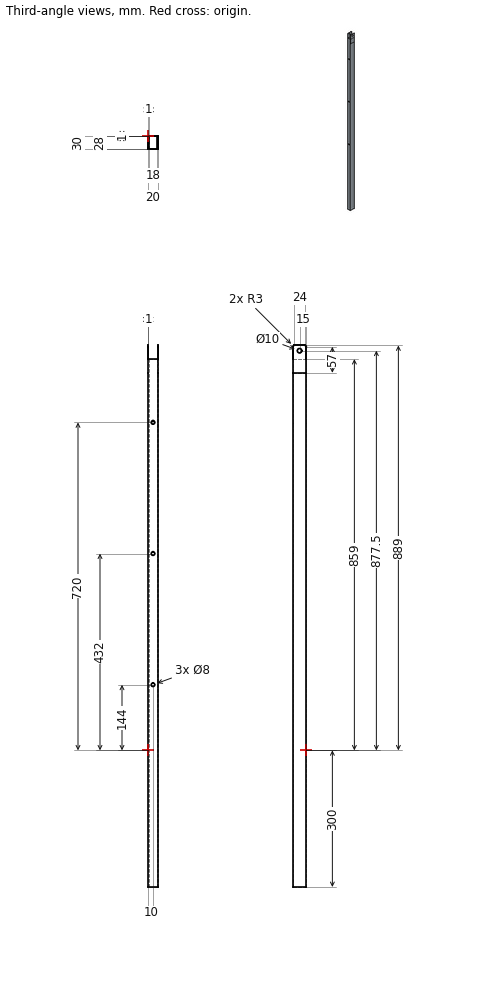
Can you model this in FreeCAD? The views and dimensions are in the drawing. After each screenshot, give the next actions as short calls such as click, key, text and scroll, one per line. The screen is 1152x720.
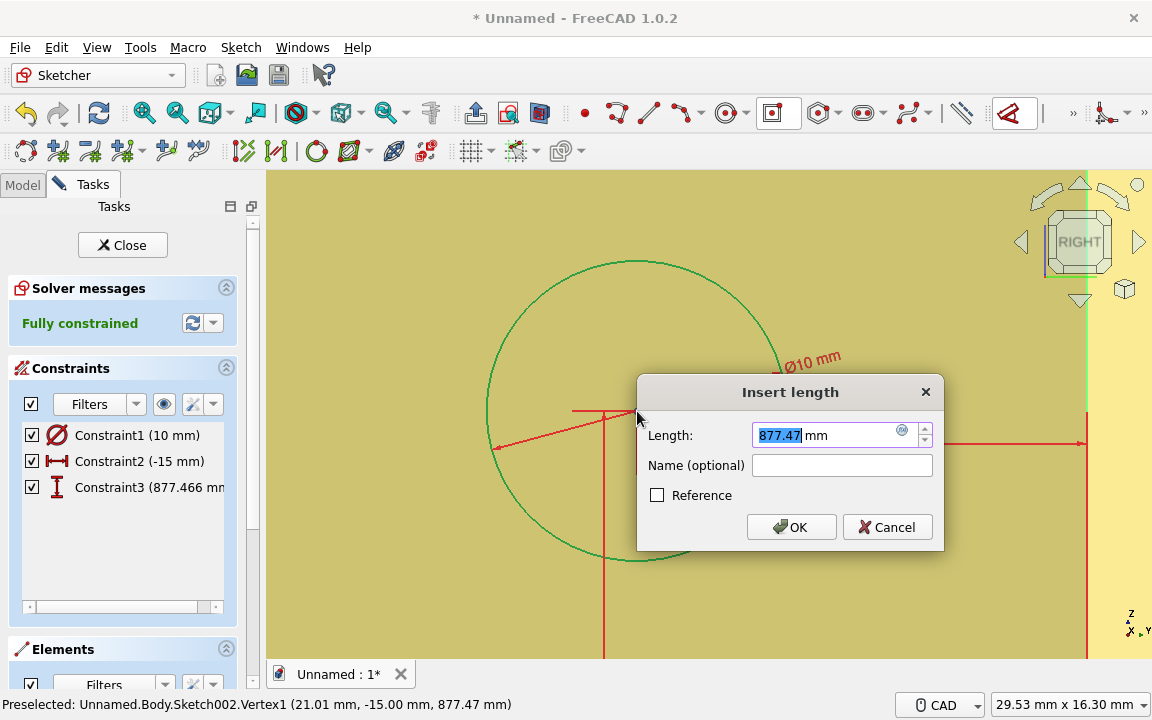
text(877.5)
key(Return)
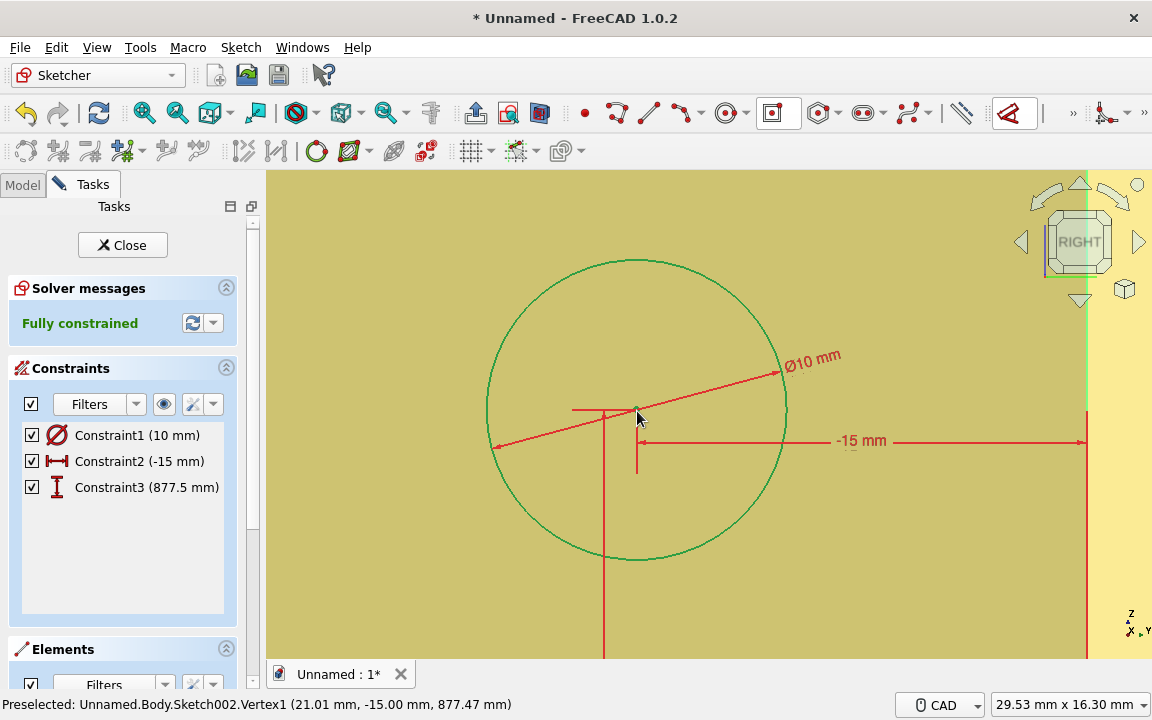
click(123, 245)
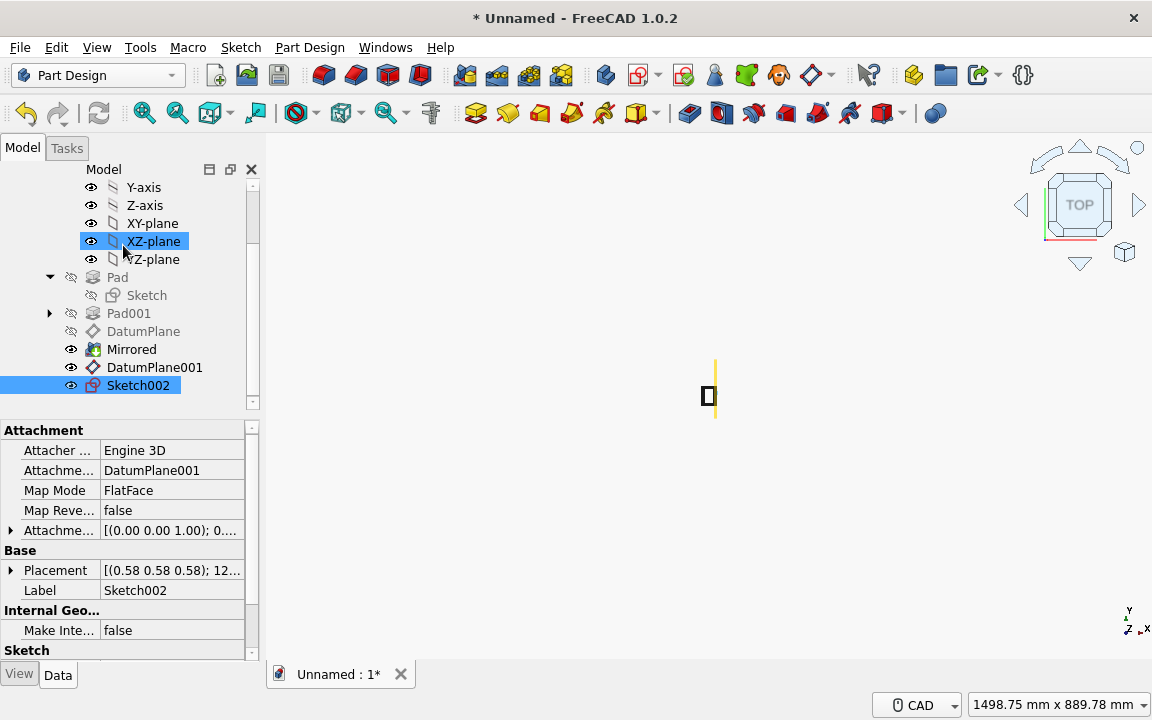
click(690, 114)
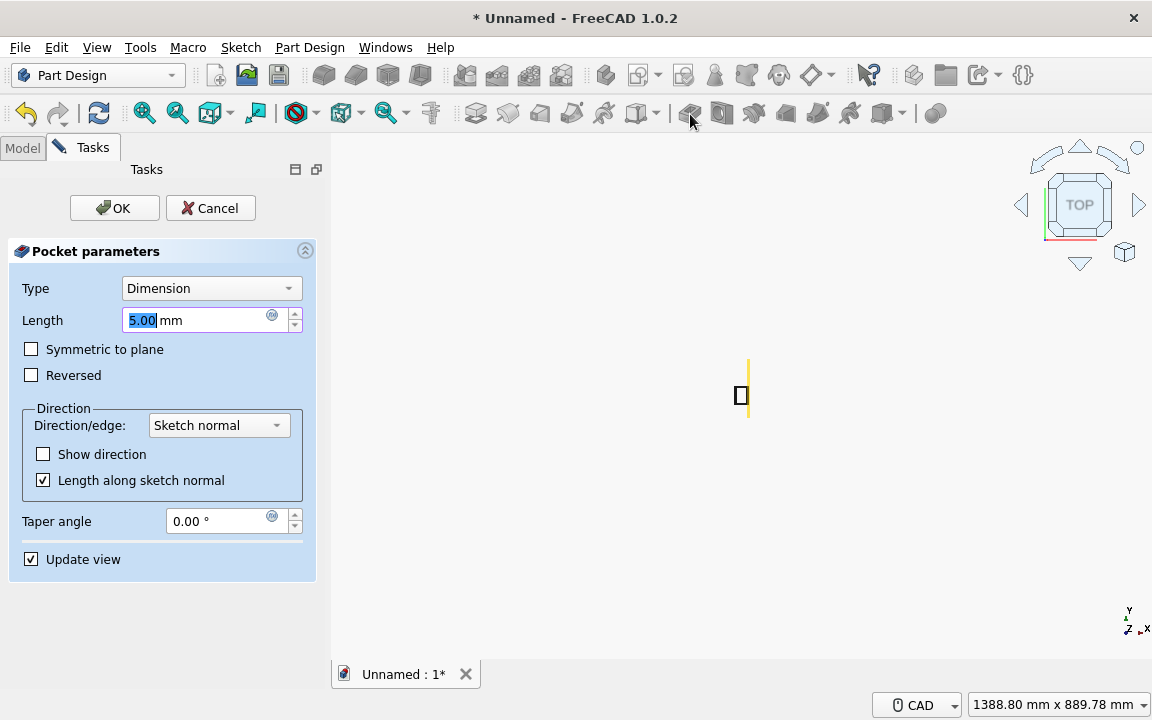
click(212, 288)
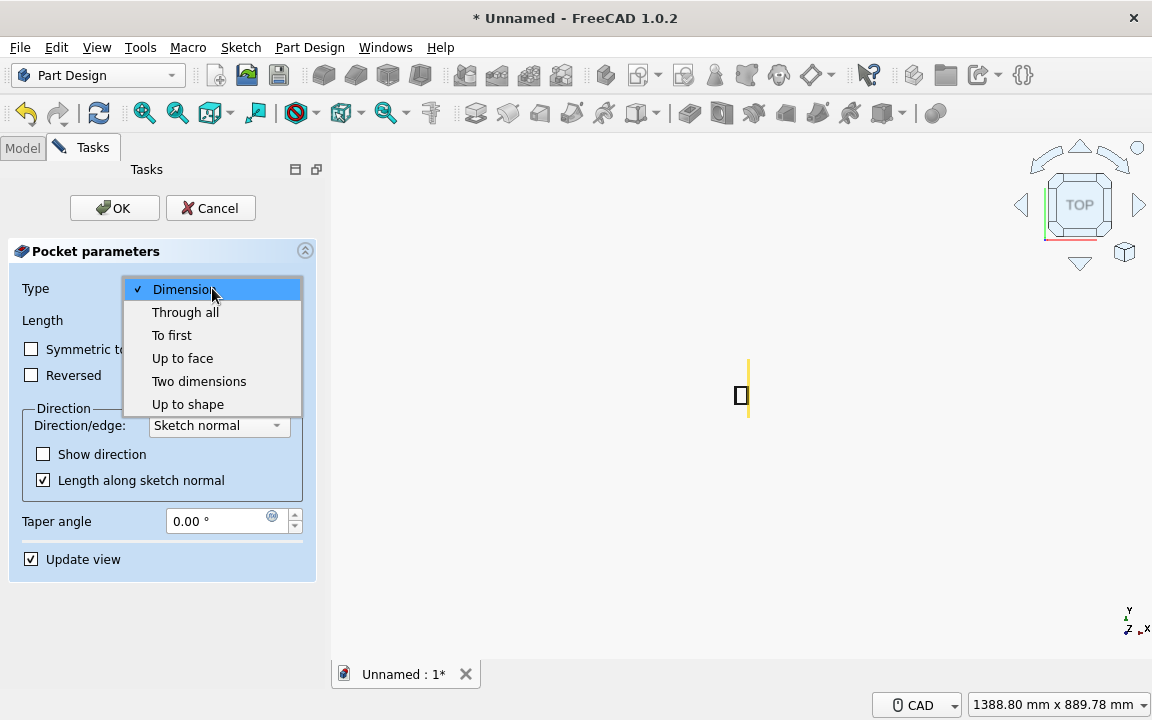
click(212, 312)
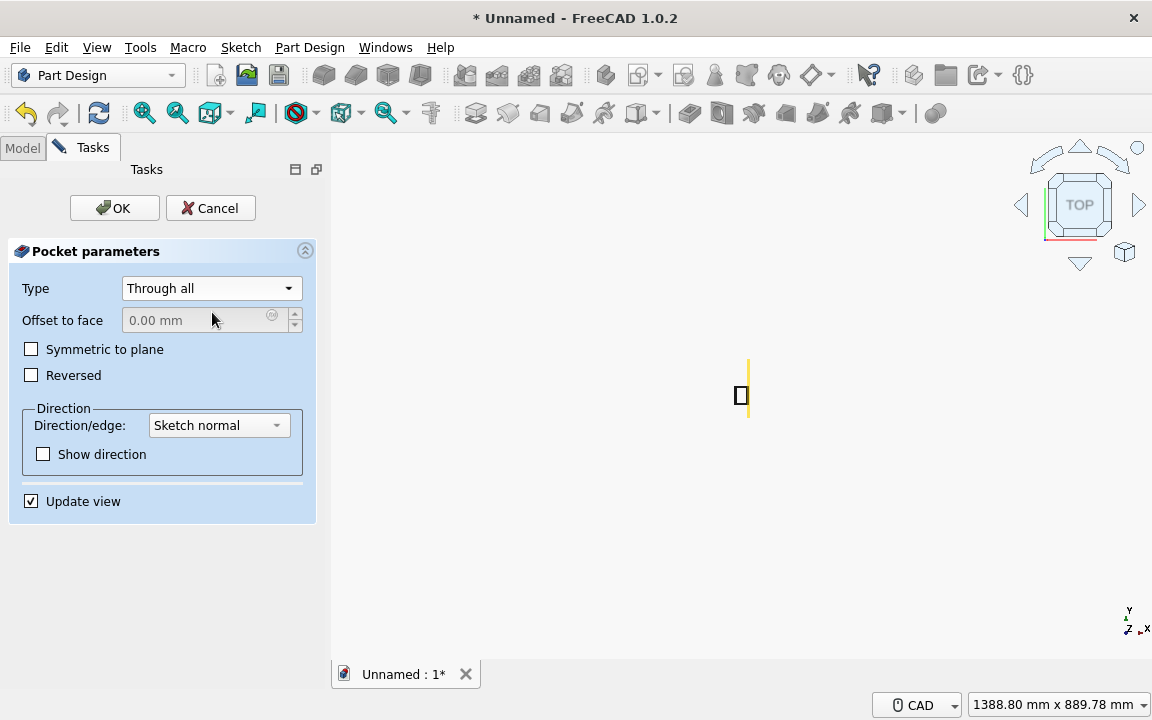
click(115, 208)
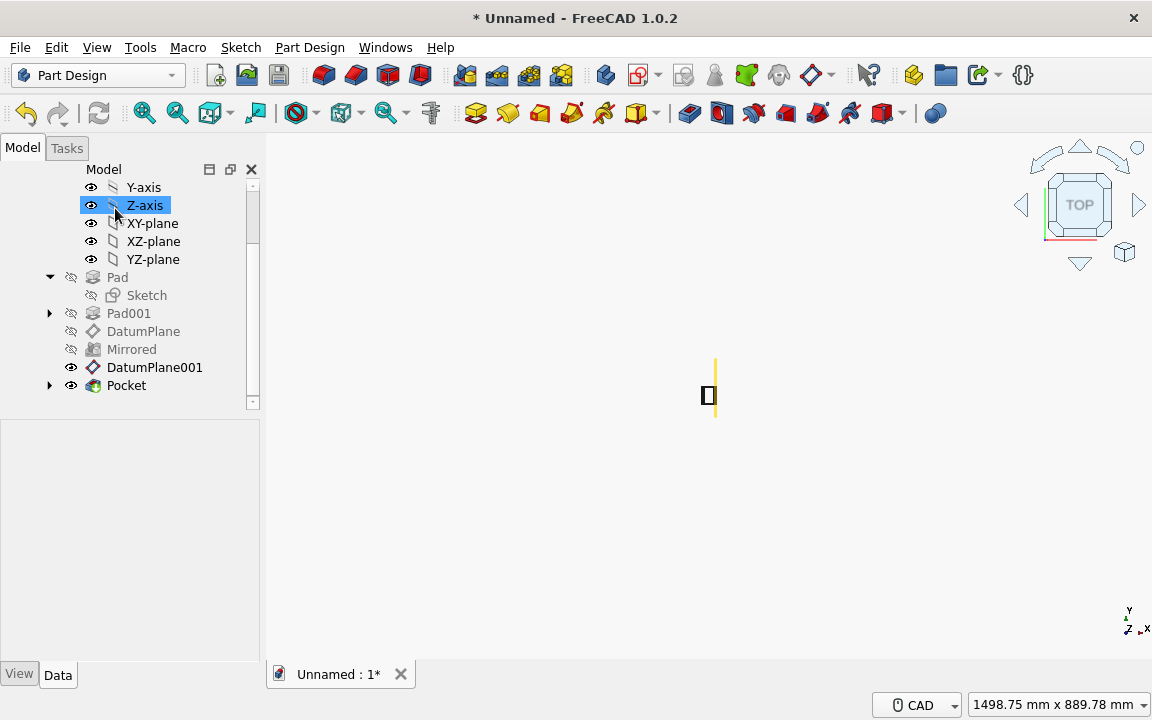
click(116, 367)
key(space)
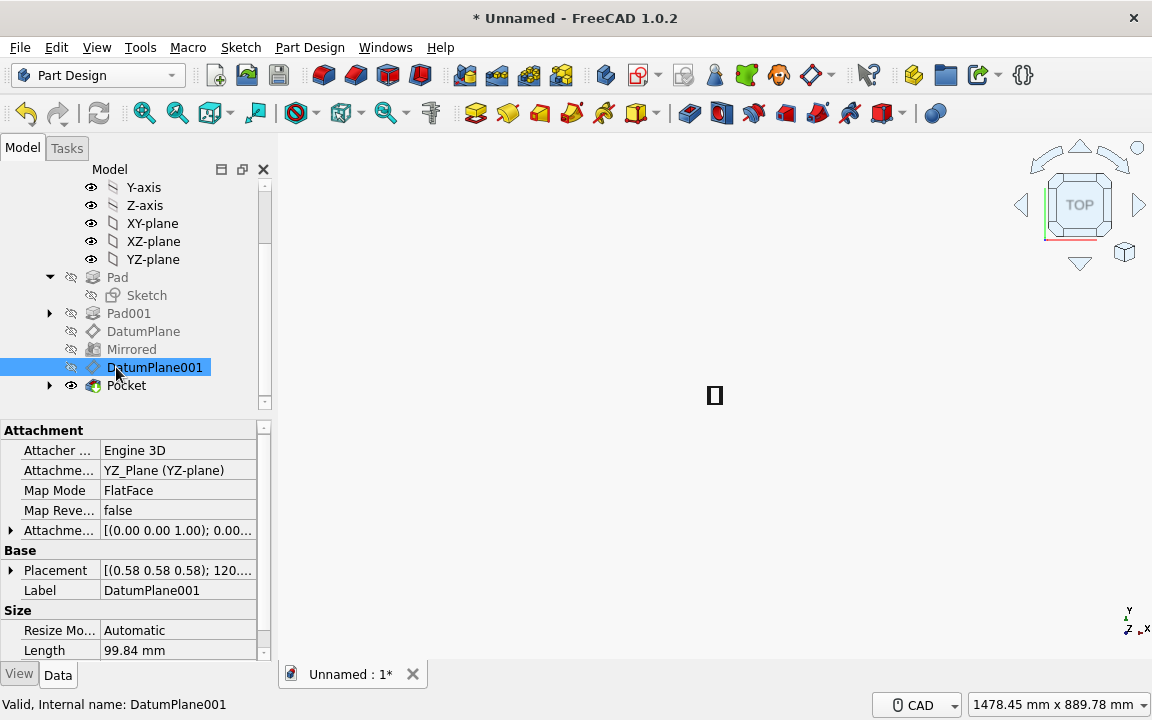
key(v)
key(f)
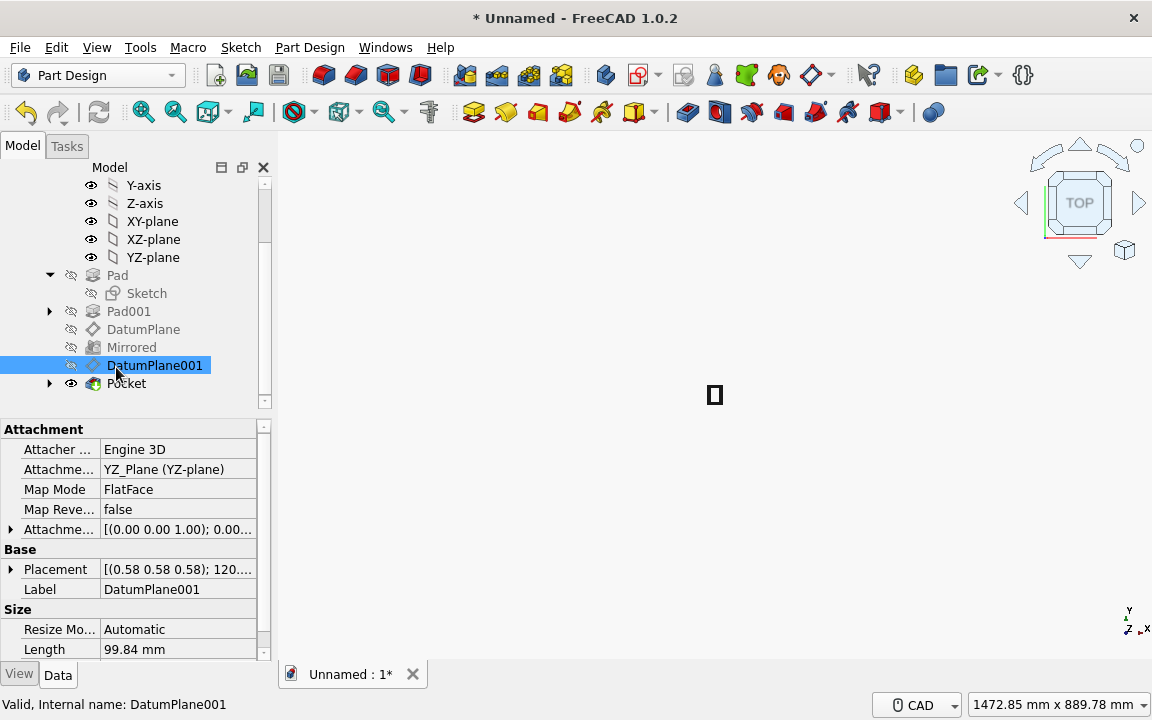
key(4)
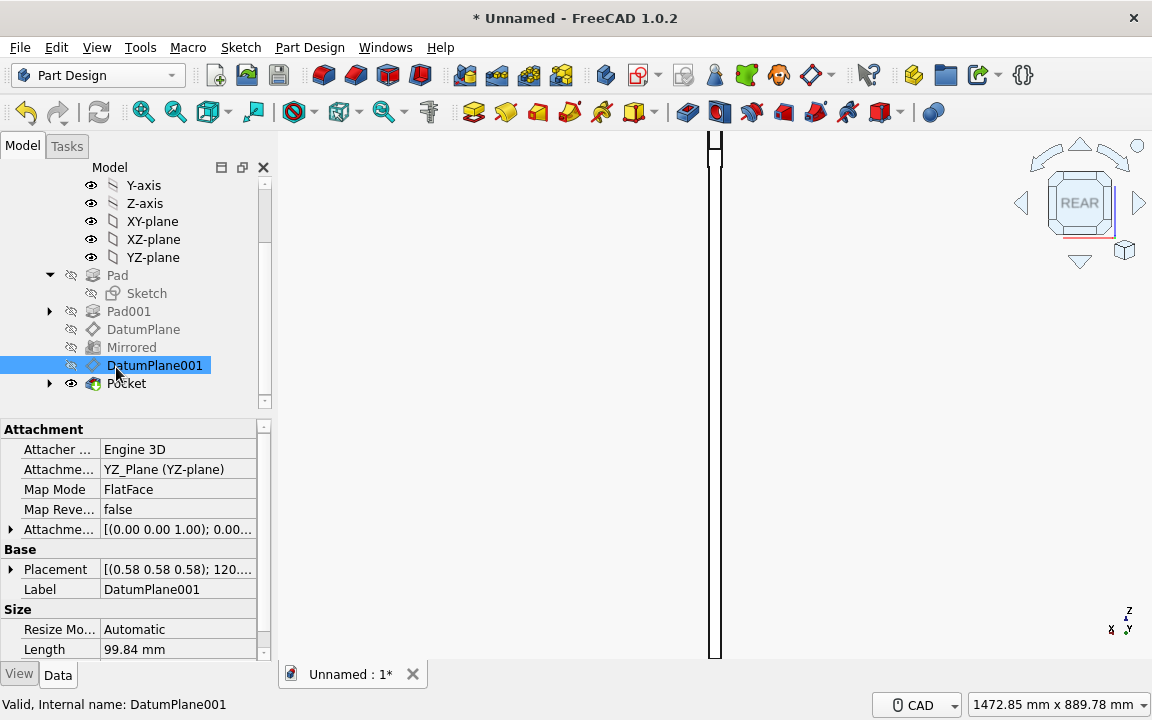
key(v)
key(f)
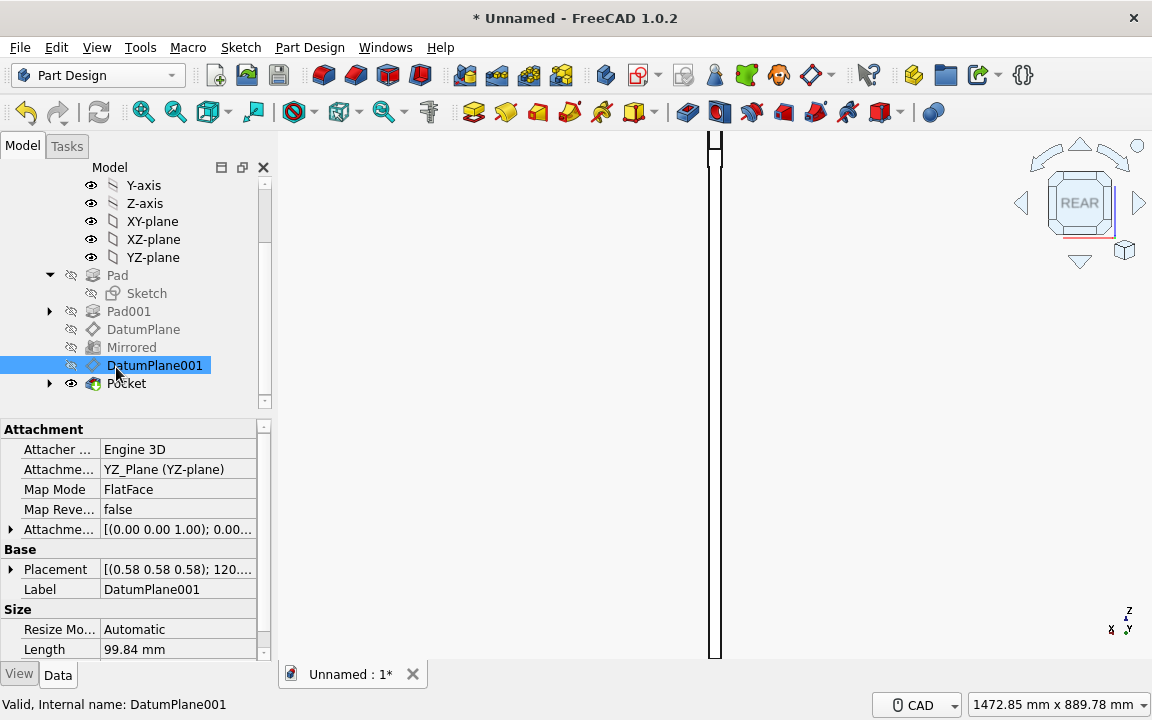
scroll(715, 170, up, 4)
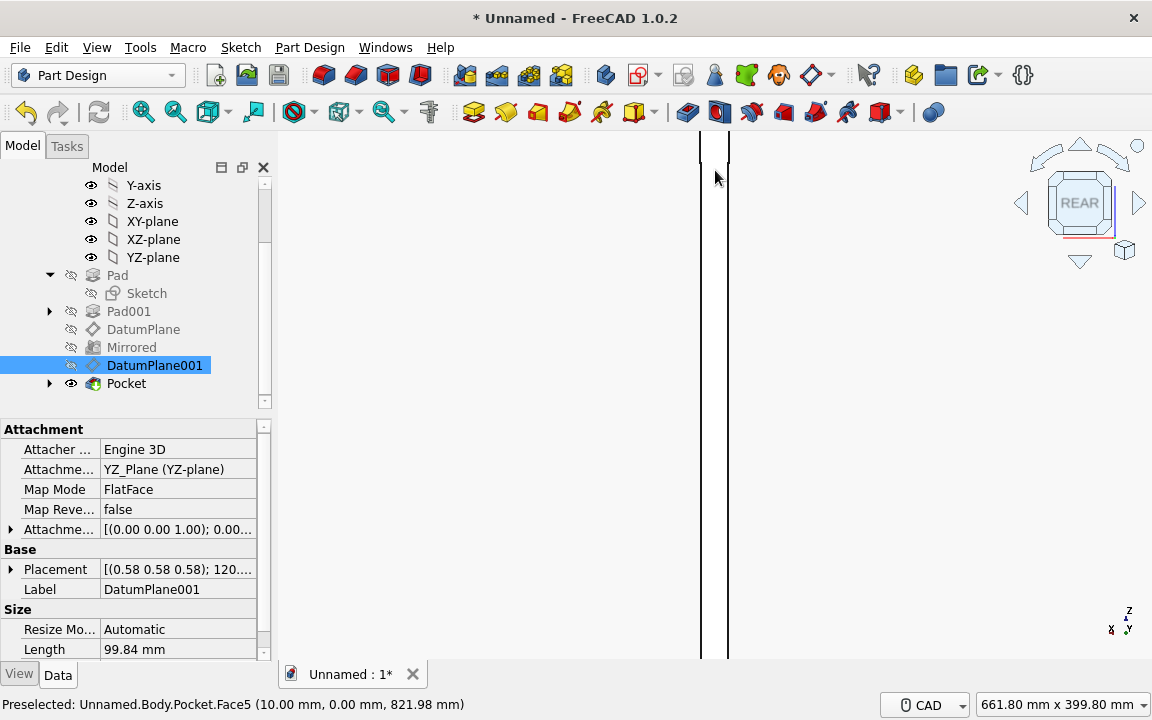
click(714, 170)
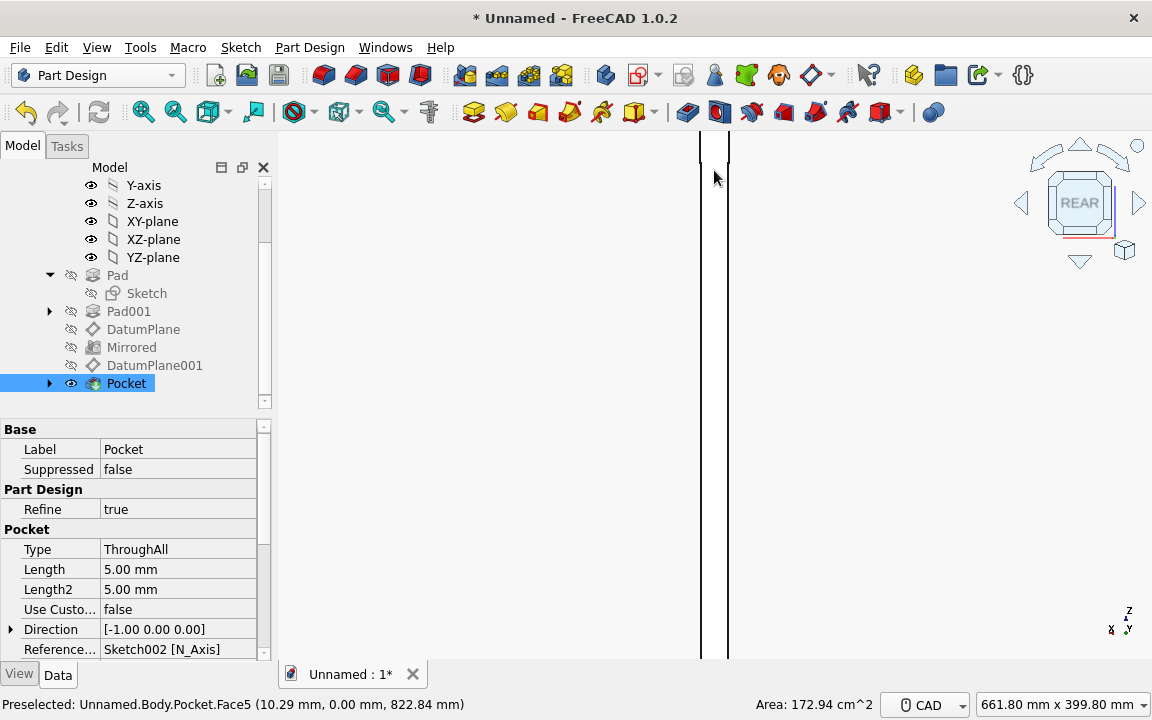
click(638, 76)